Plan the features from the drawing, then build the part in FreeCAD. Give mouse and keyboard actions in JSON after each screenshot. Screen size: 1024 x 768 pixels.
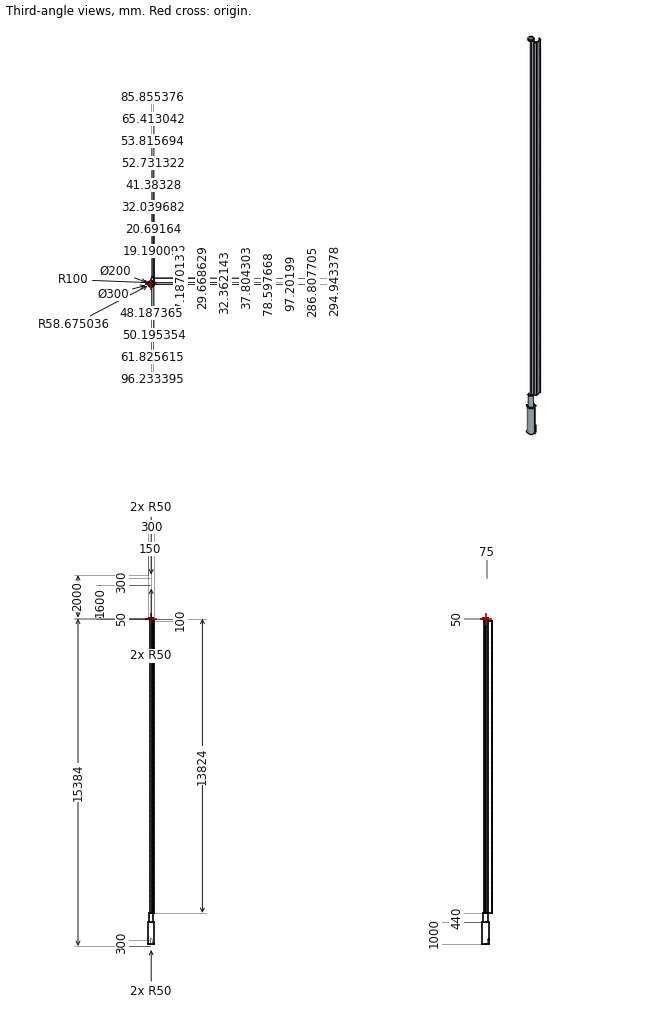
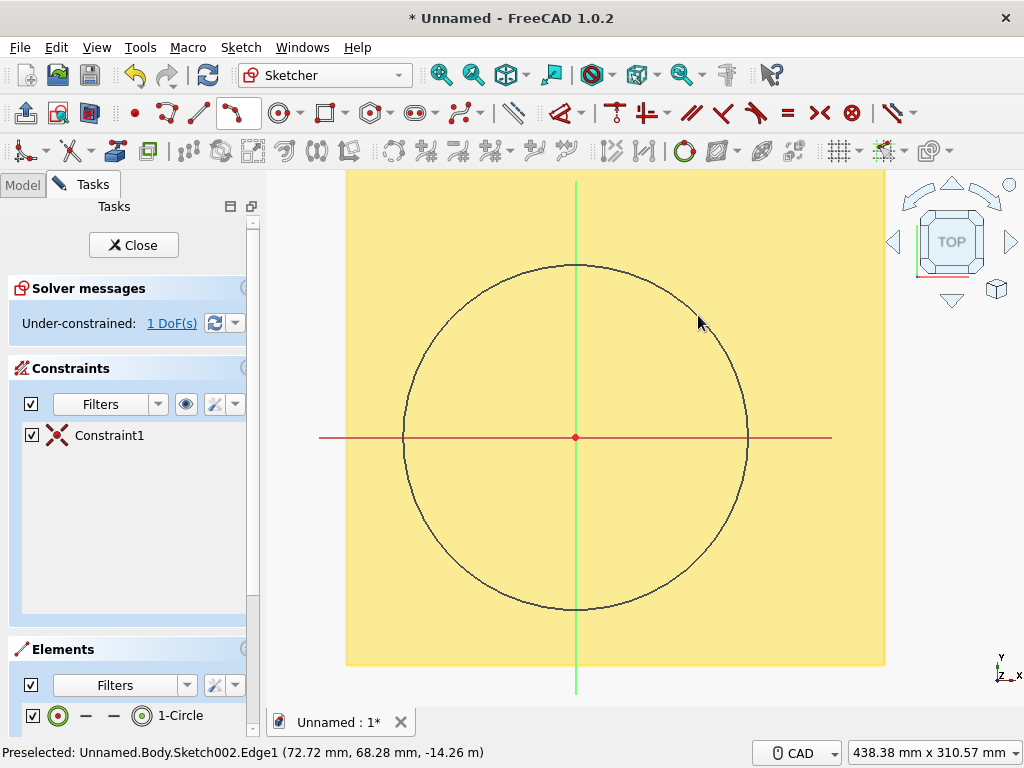
{"action": "left_click", "coordinate": [560, 114]}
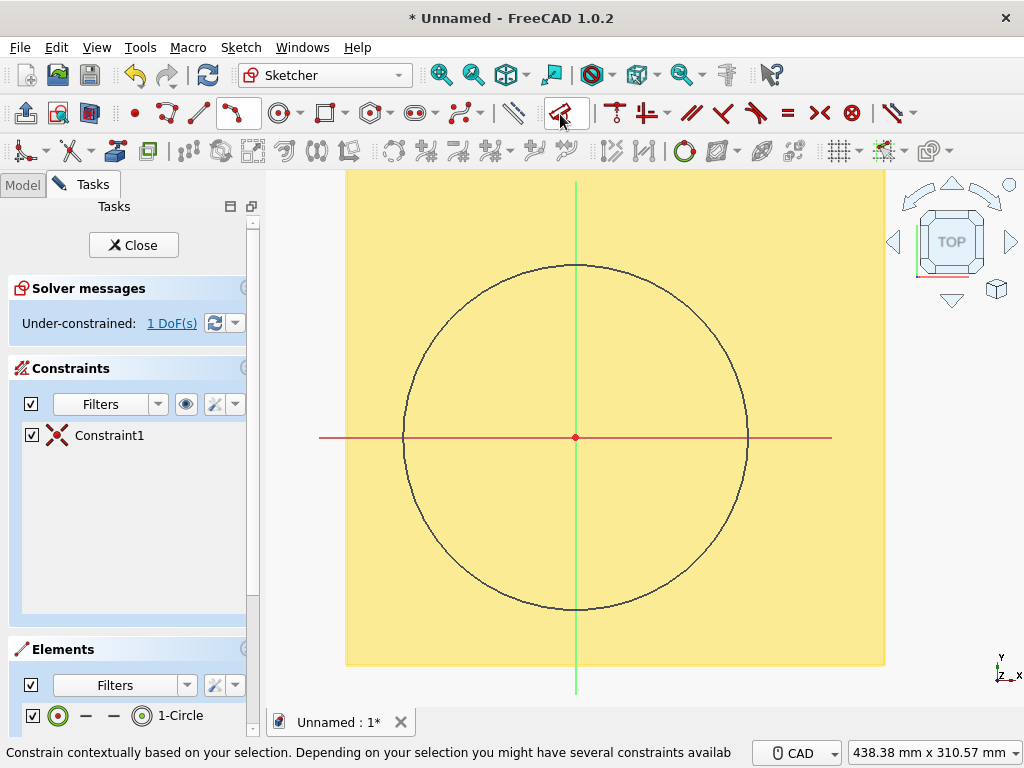
{"action": "left_click", "coordinate": [697, 315]}
{"action": "left_click", "coordinate": [720, 292]}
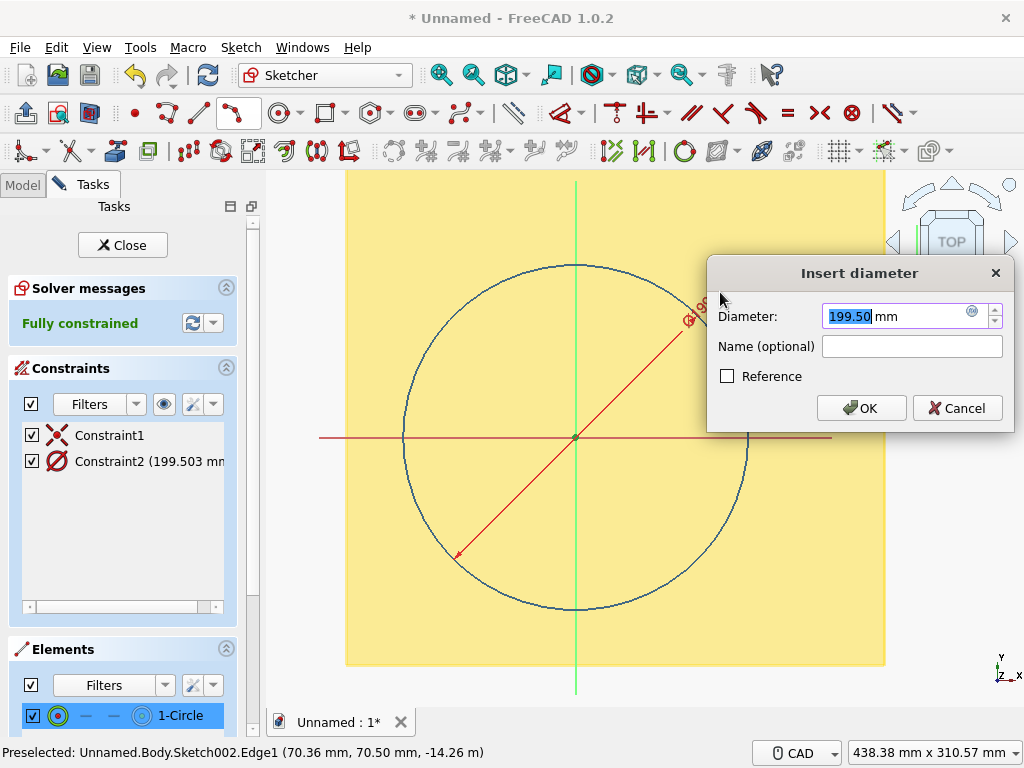
{"action": "type", "text": "200"}
{"action": "key", "text": "Return"}
{"action": "key", "text": "Escape"}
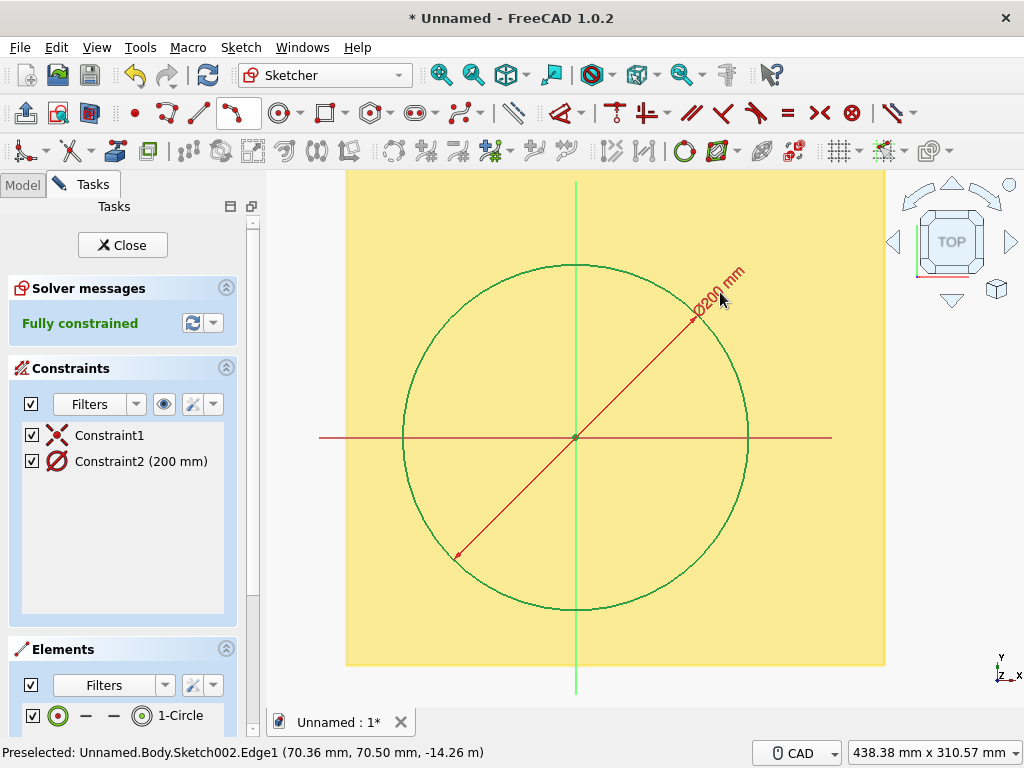
{"action": "left_click", "coordinate": [123, 245]}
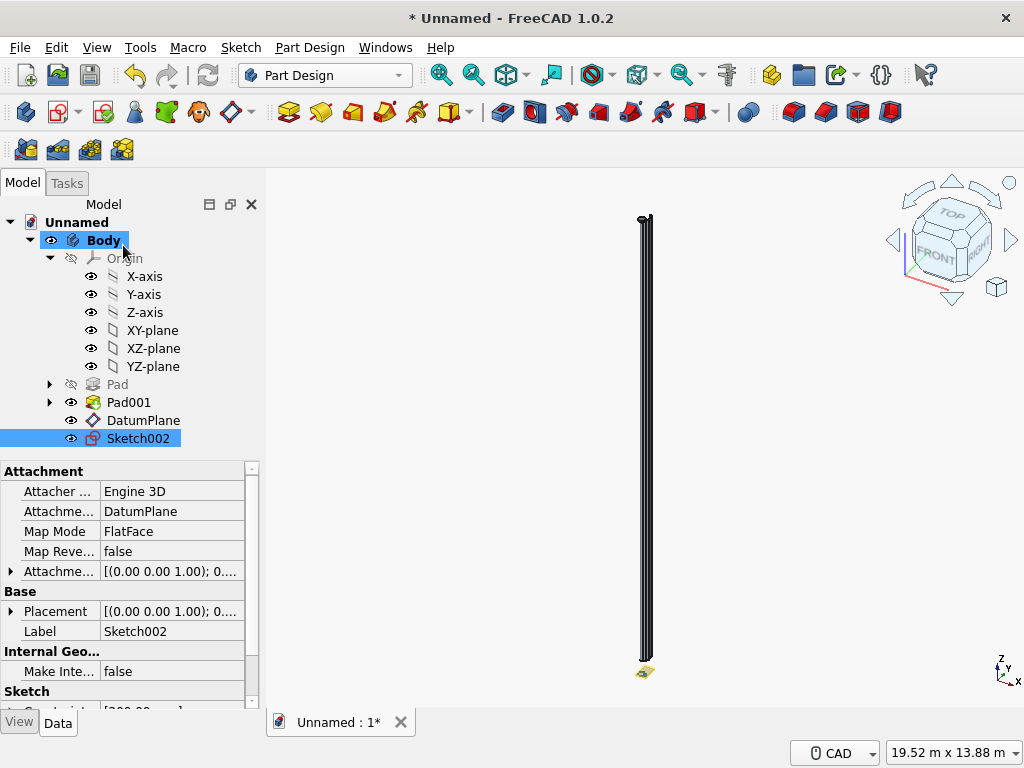
{"action": "left_click", "coordinate": [290, 112]}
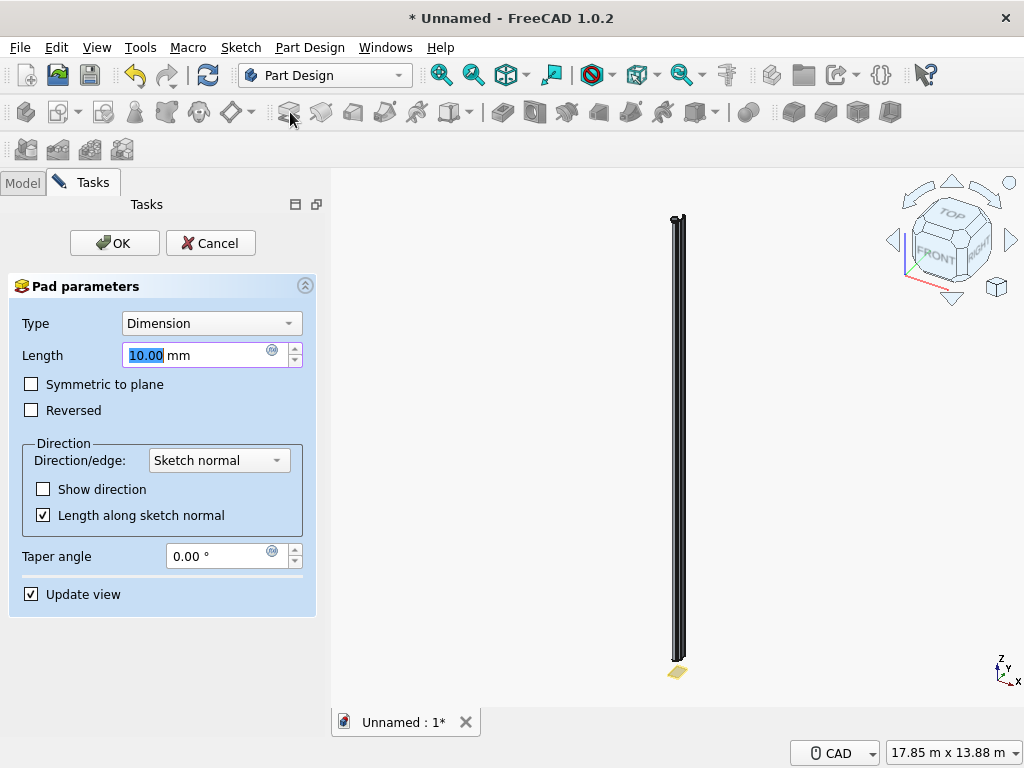
{"action": "type", "text": "440"}
{"action": "key", "text": "Tab"}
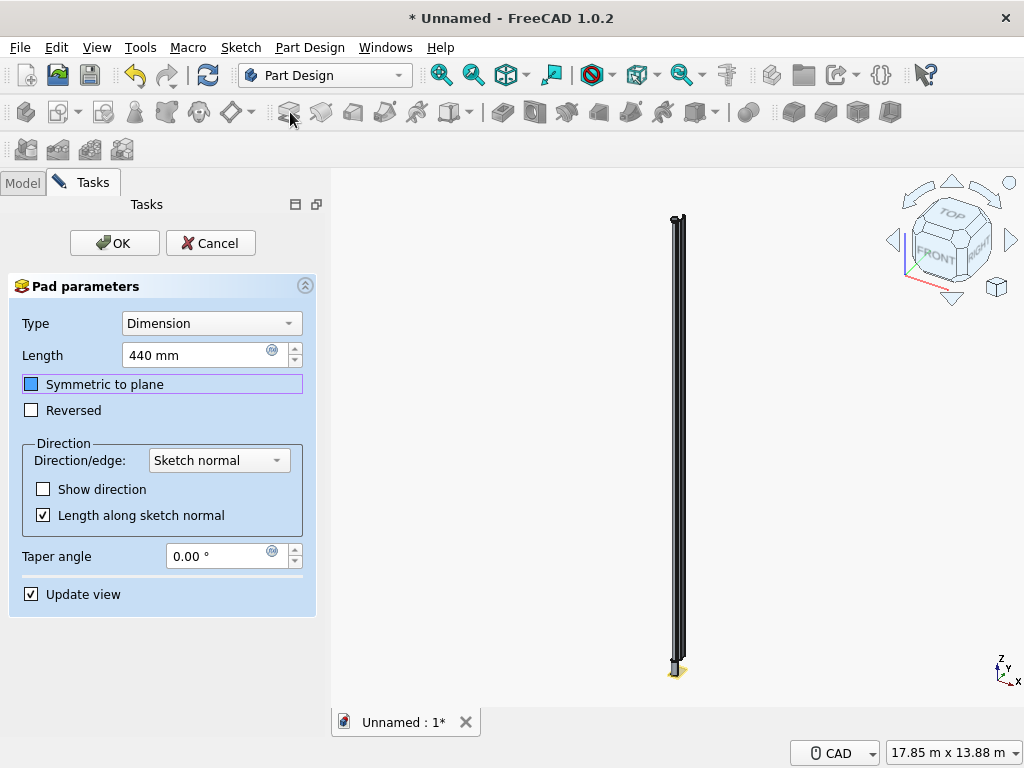
{"action": "left_click", "coordinate": [115, 243]}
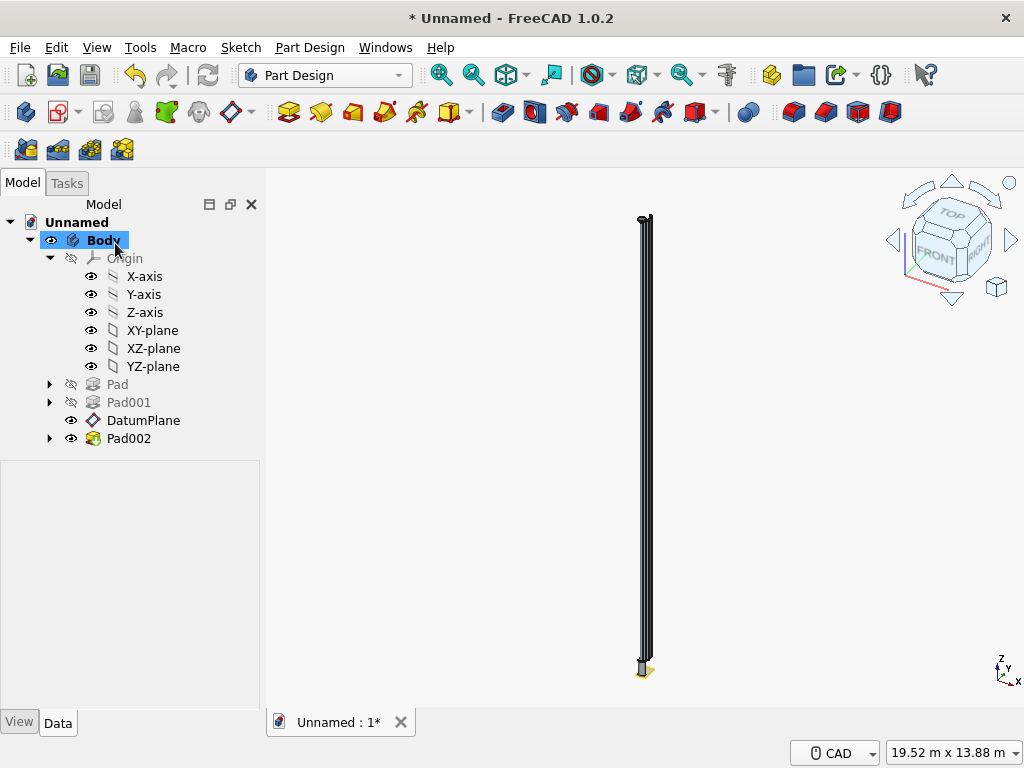
{"action": "left_click", "coordinate": [116, 420]}
{"action": "key", "text": "space"}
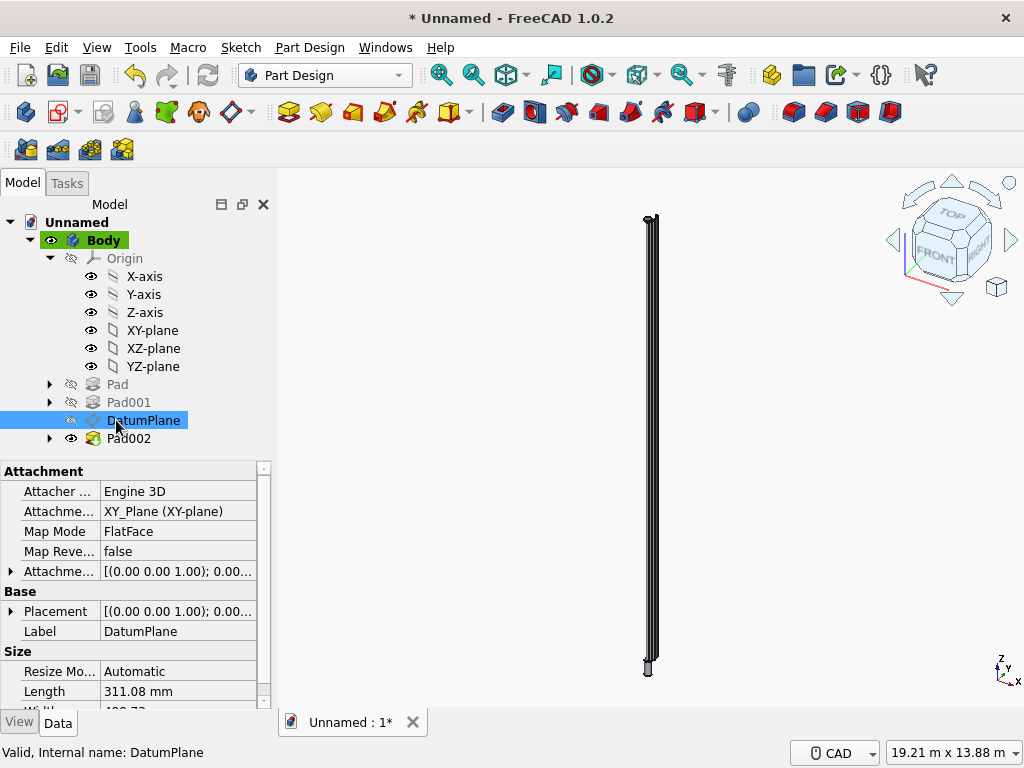
{"action": "left_click", "coordinate": [136, 330]}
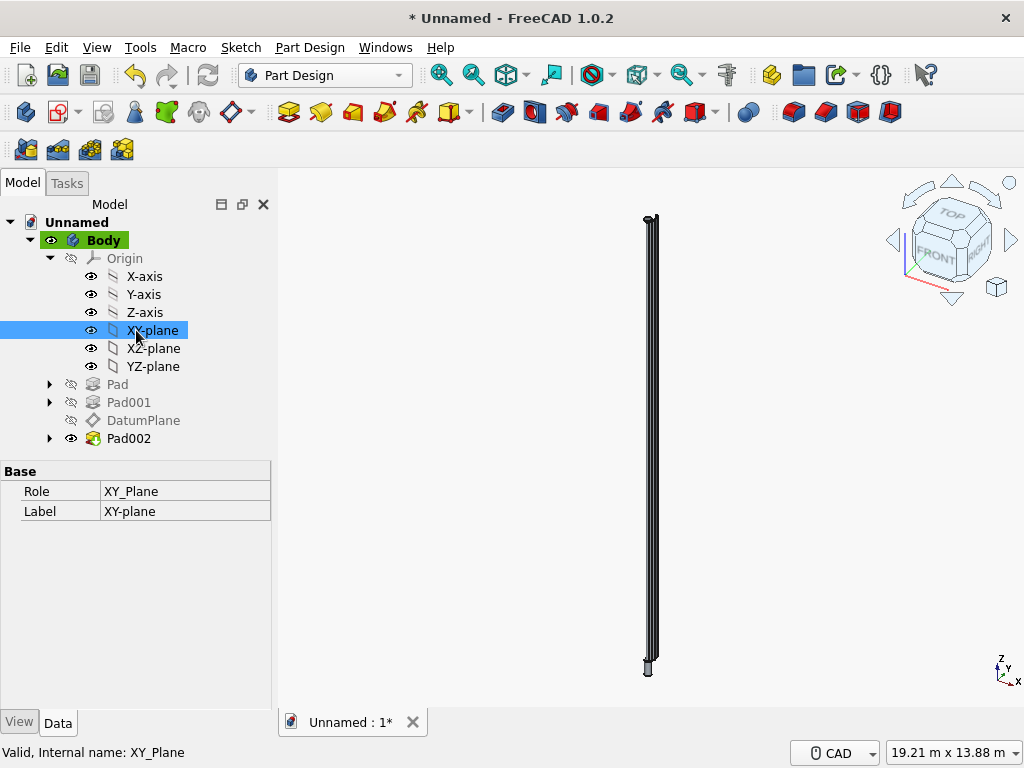
{"action": "left_click", "coordinate": [232, 112]}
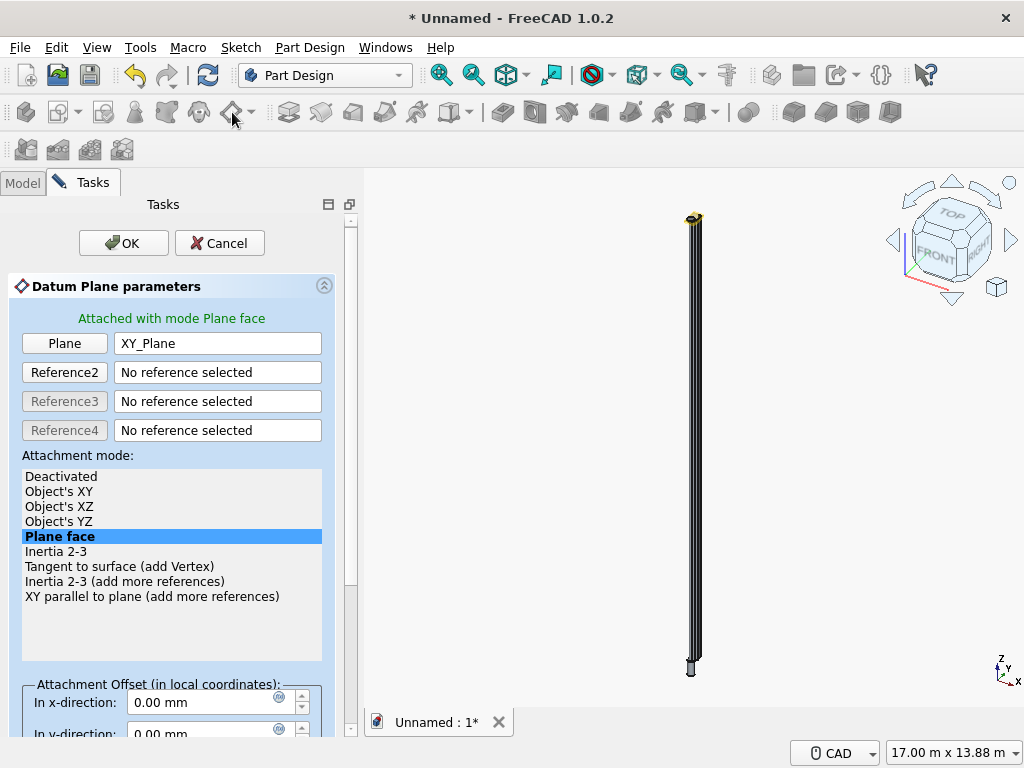
{"action": "scroll", "coordinate": [351, 475], "scroll_direction": "down", "scroll_amount": 2}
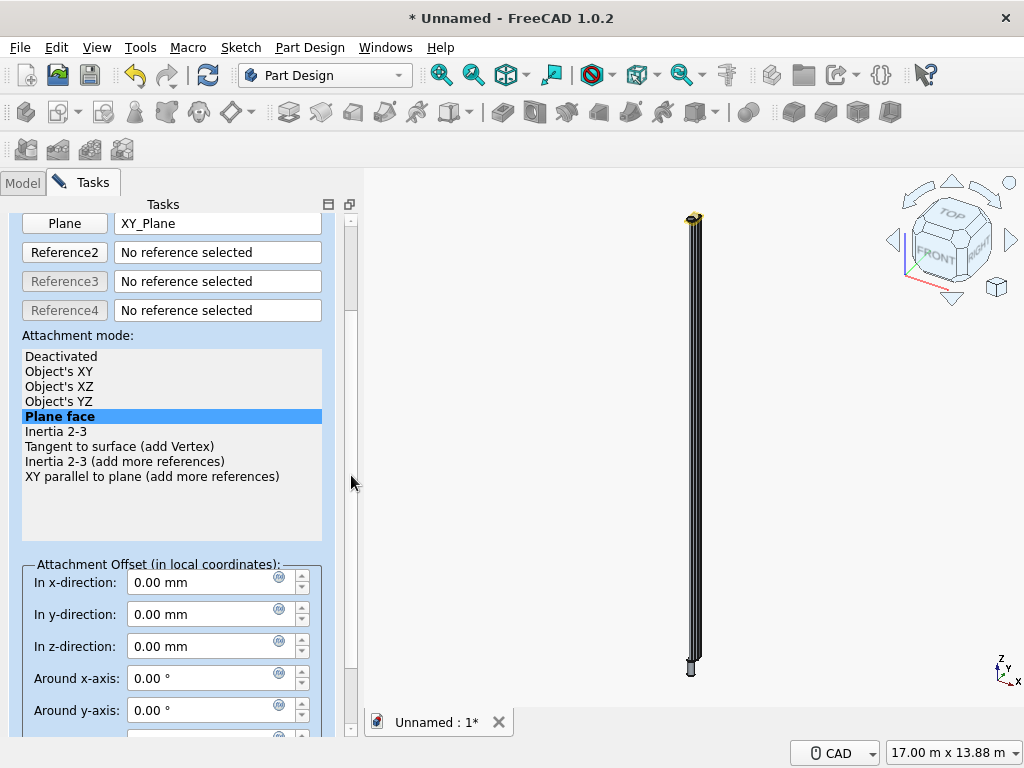
{"action": "triple_click", "coordinate": [210, 646]}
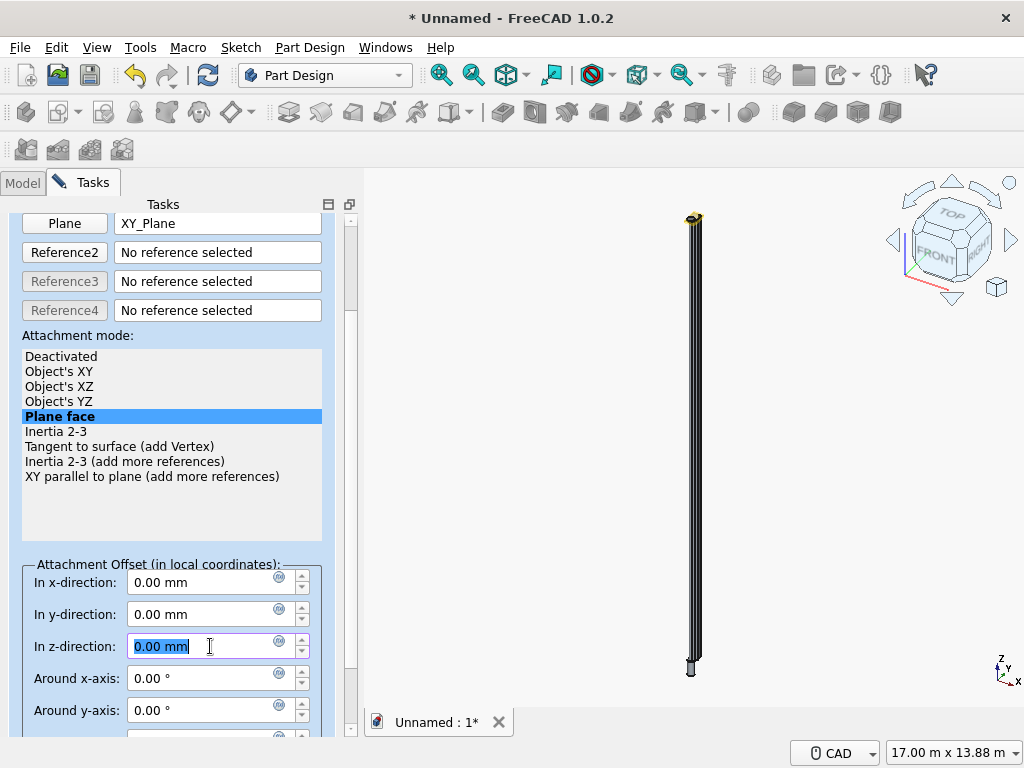
{"action": "type", "text": "-100"}
{"action": "key", "text": "Tab"}